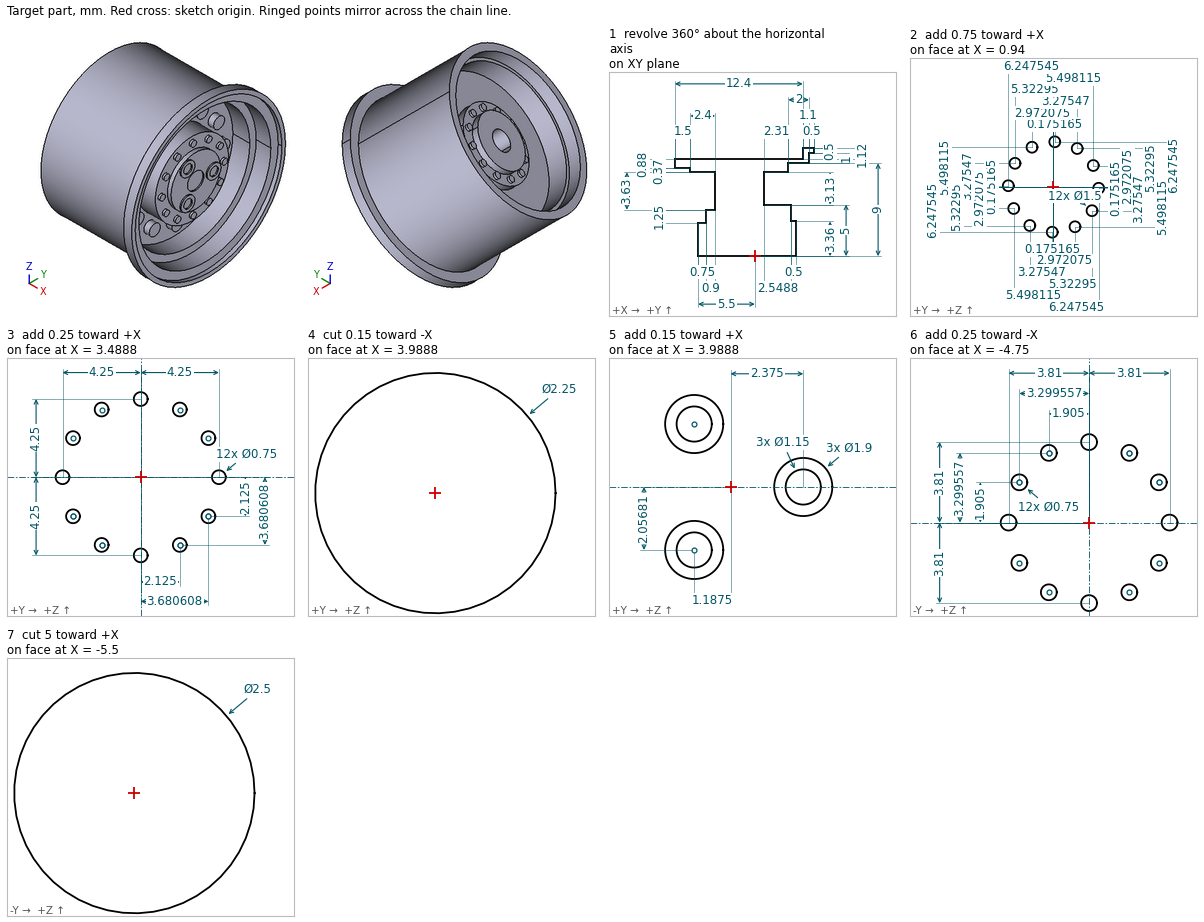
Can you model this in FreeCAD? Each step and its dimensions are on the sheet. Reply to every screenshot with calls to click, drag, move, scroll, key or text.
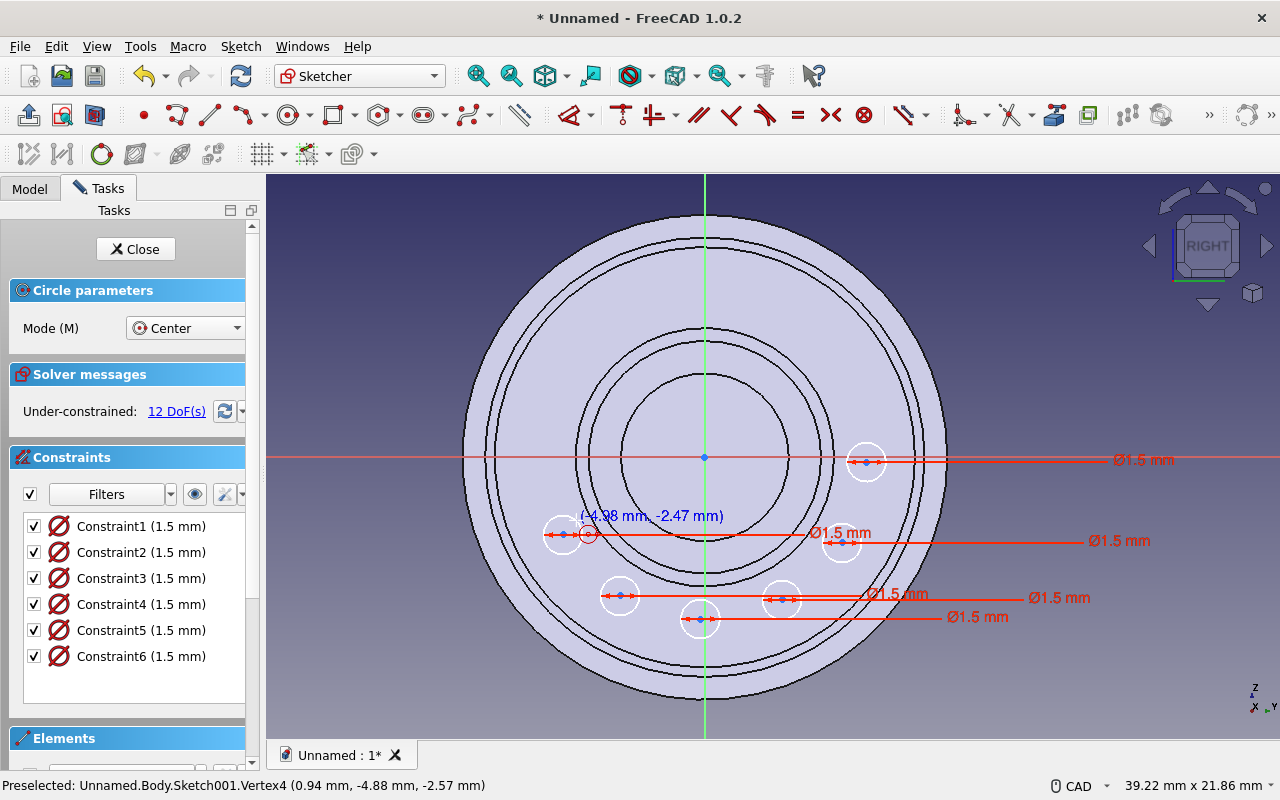
scroll(543, 453, up, 7)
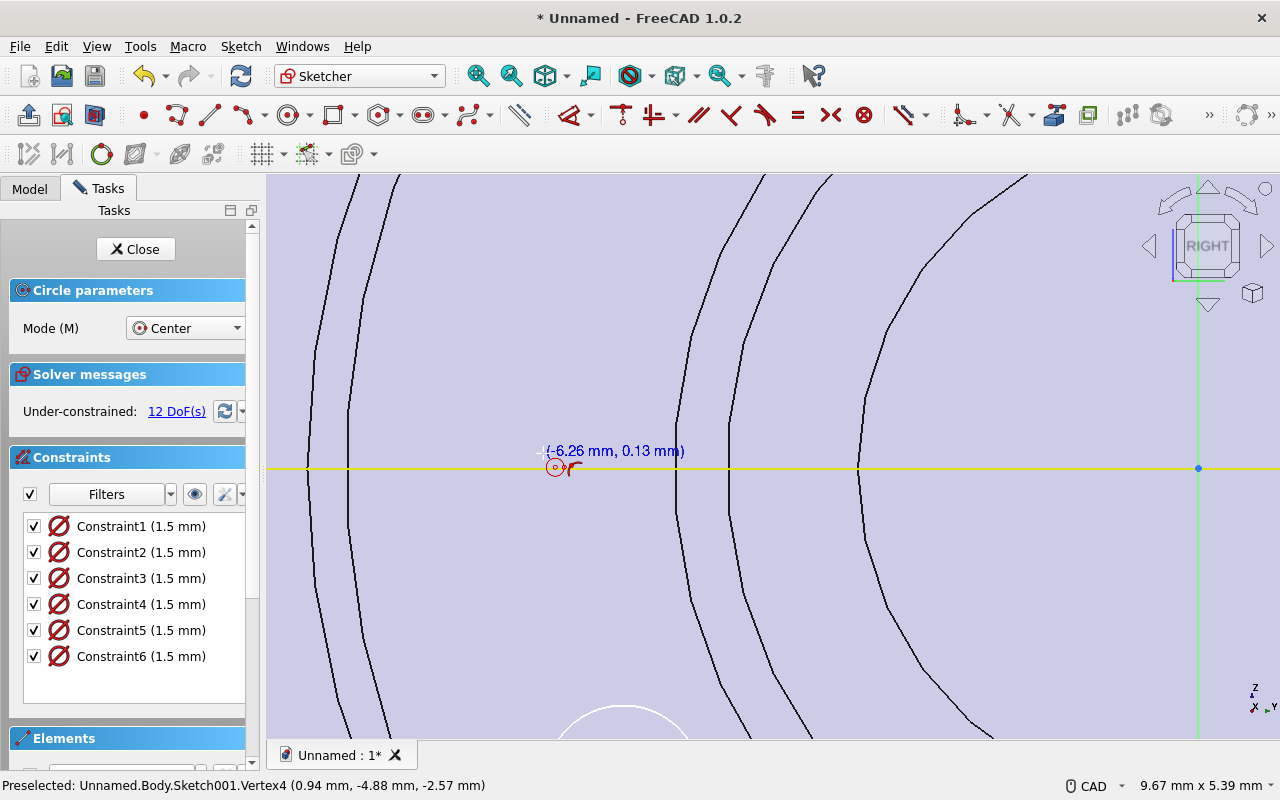
click(544, 450)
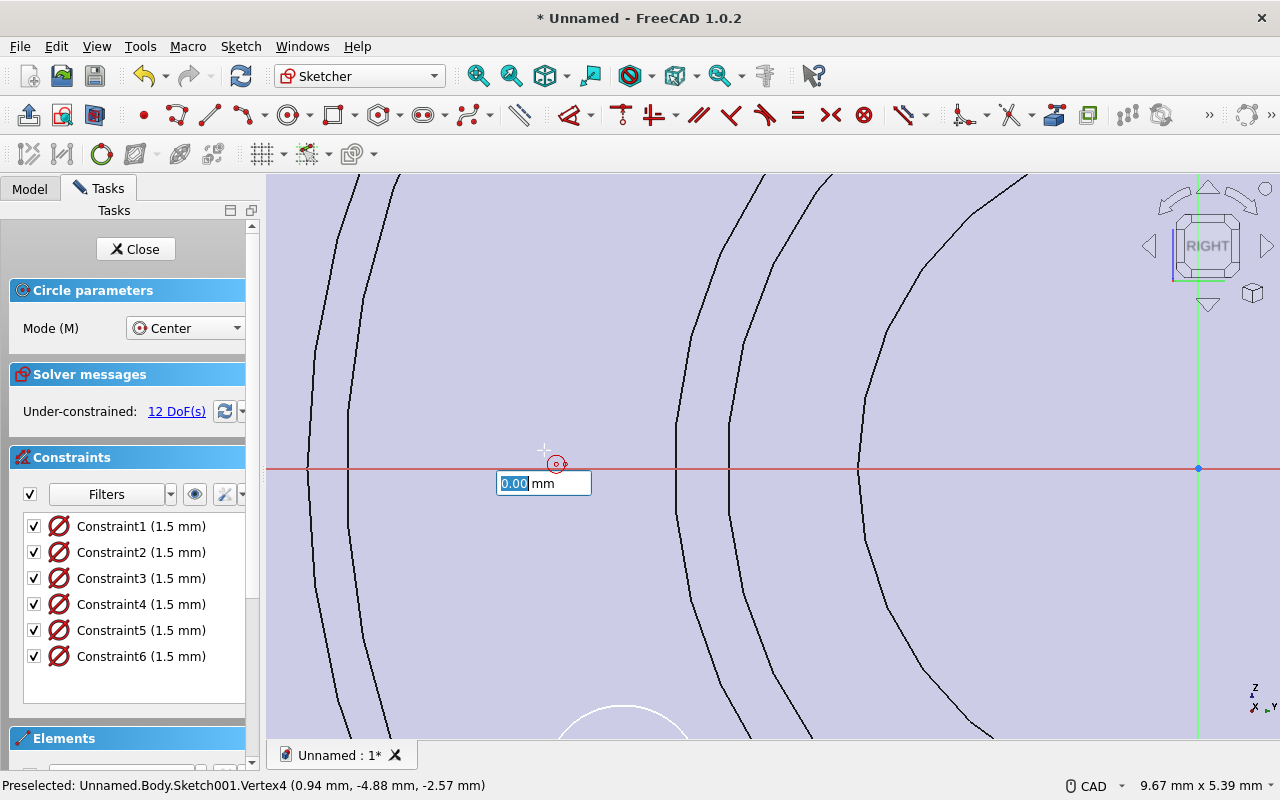
scroll(543, 452, down, 7)
move(557, 438)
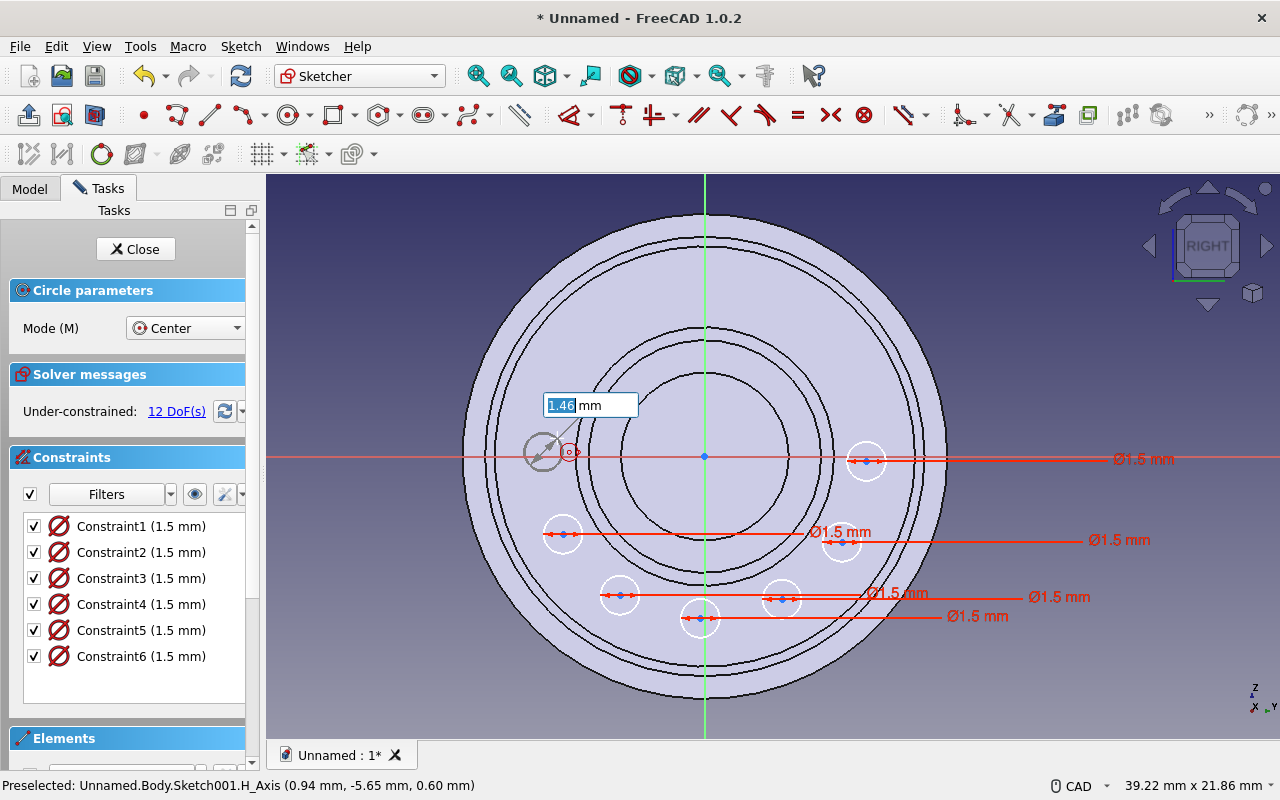
text(1.5)
key(Return)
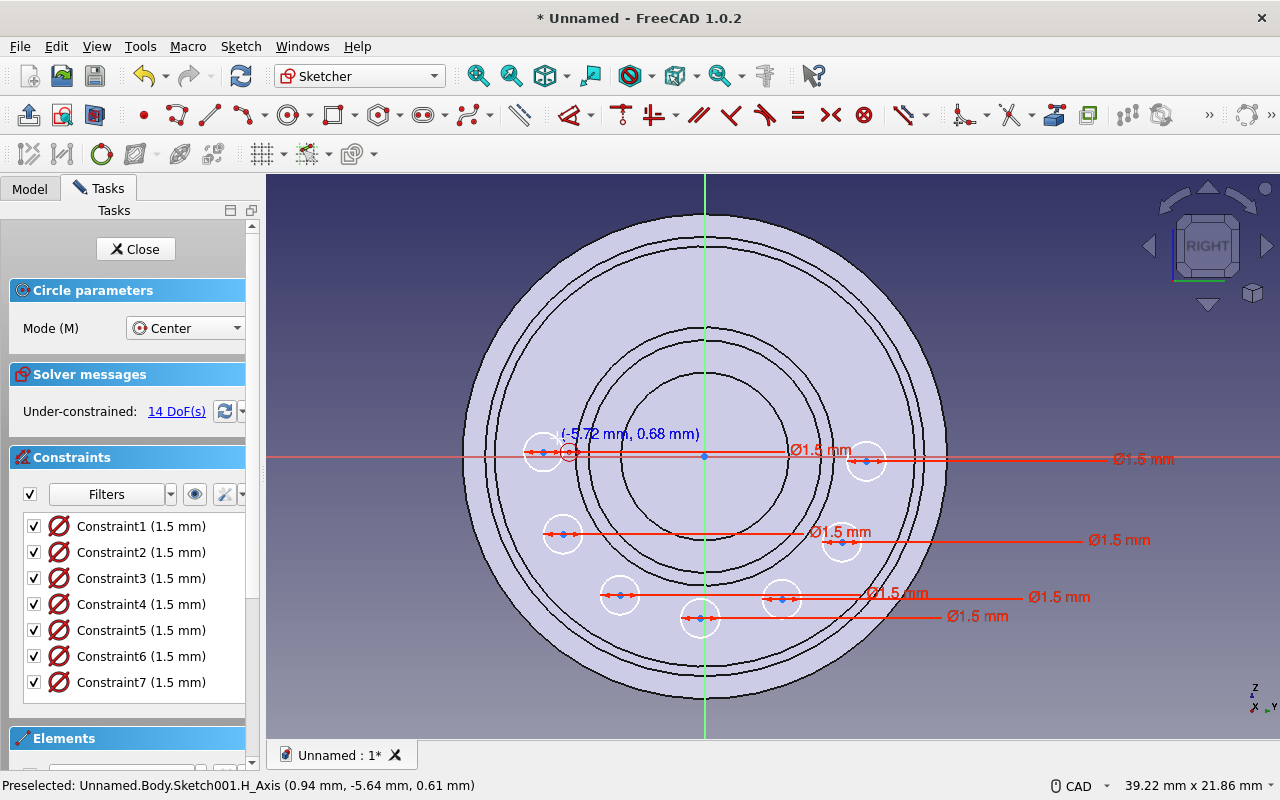
click(567, 372)
move(581, 358)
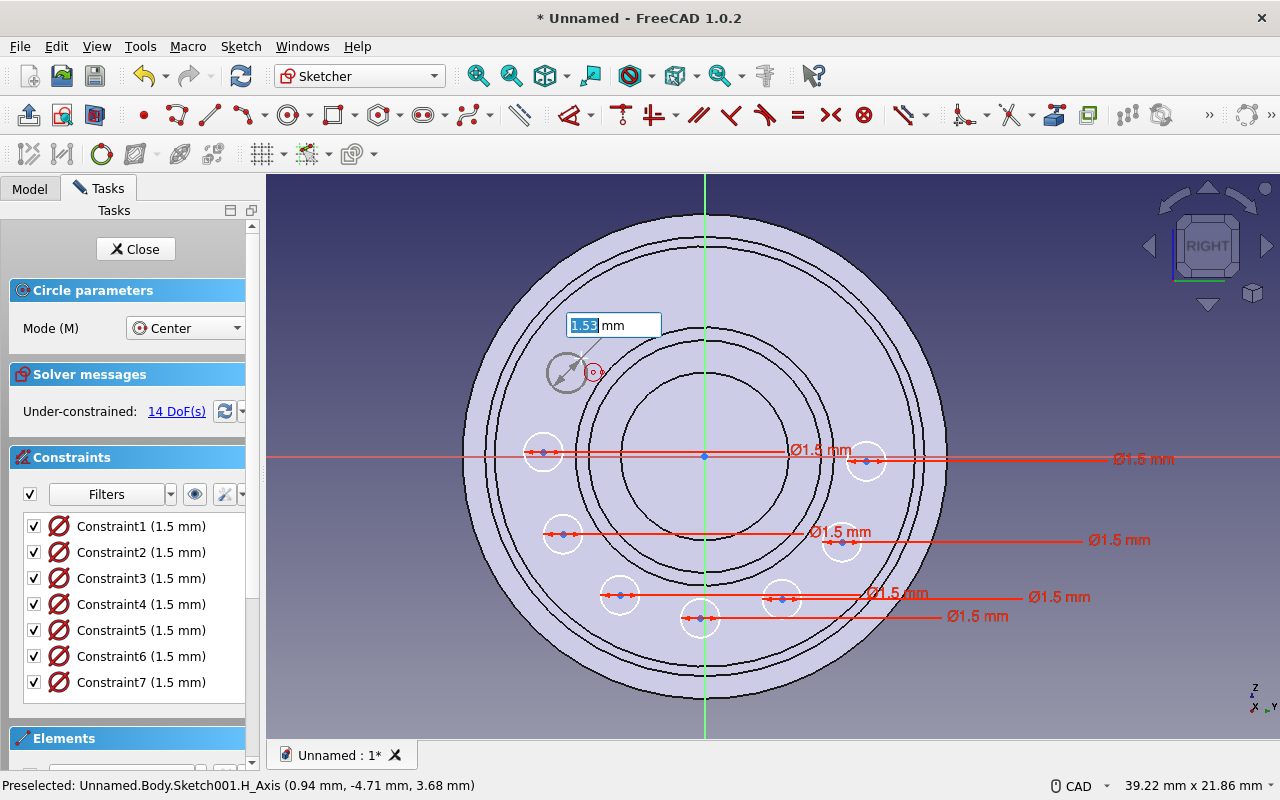
text(1.5)
key(Return)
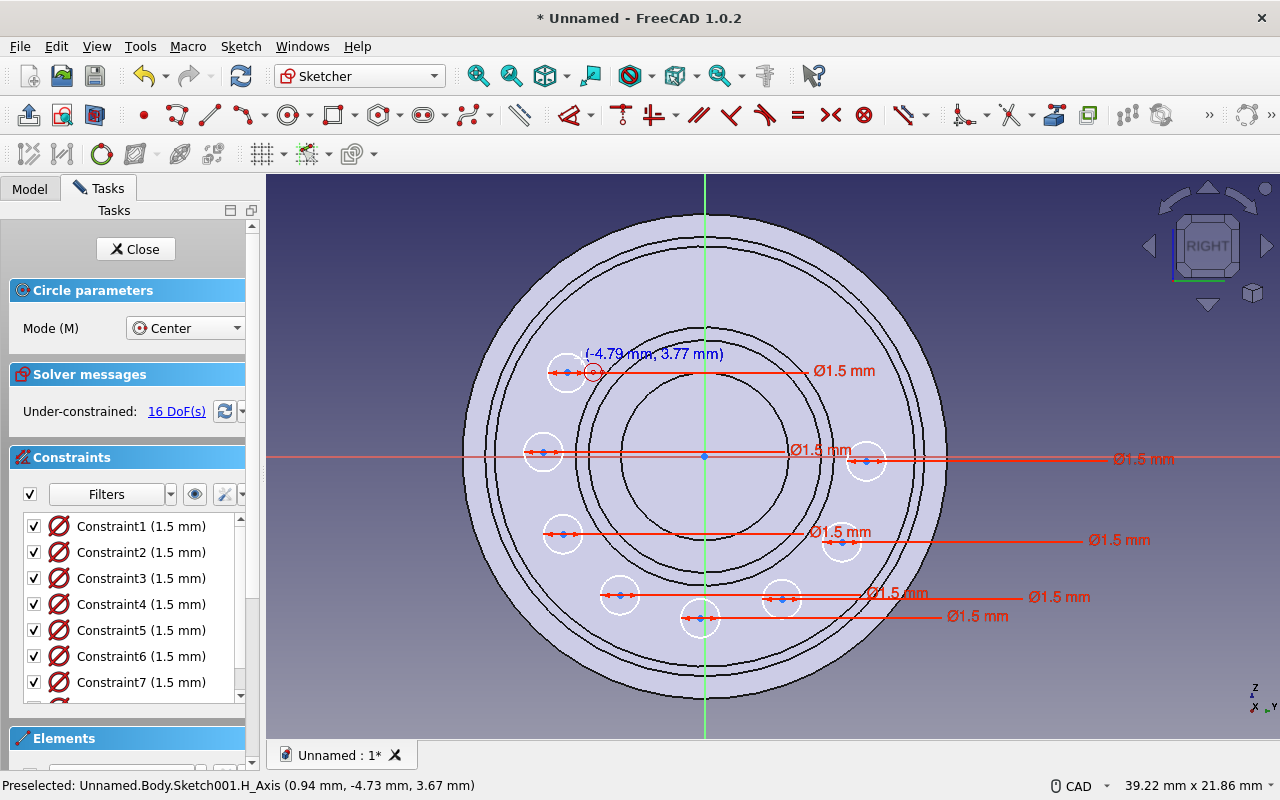
click(628, 314)
move(642, 301)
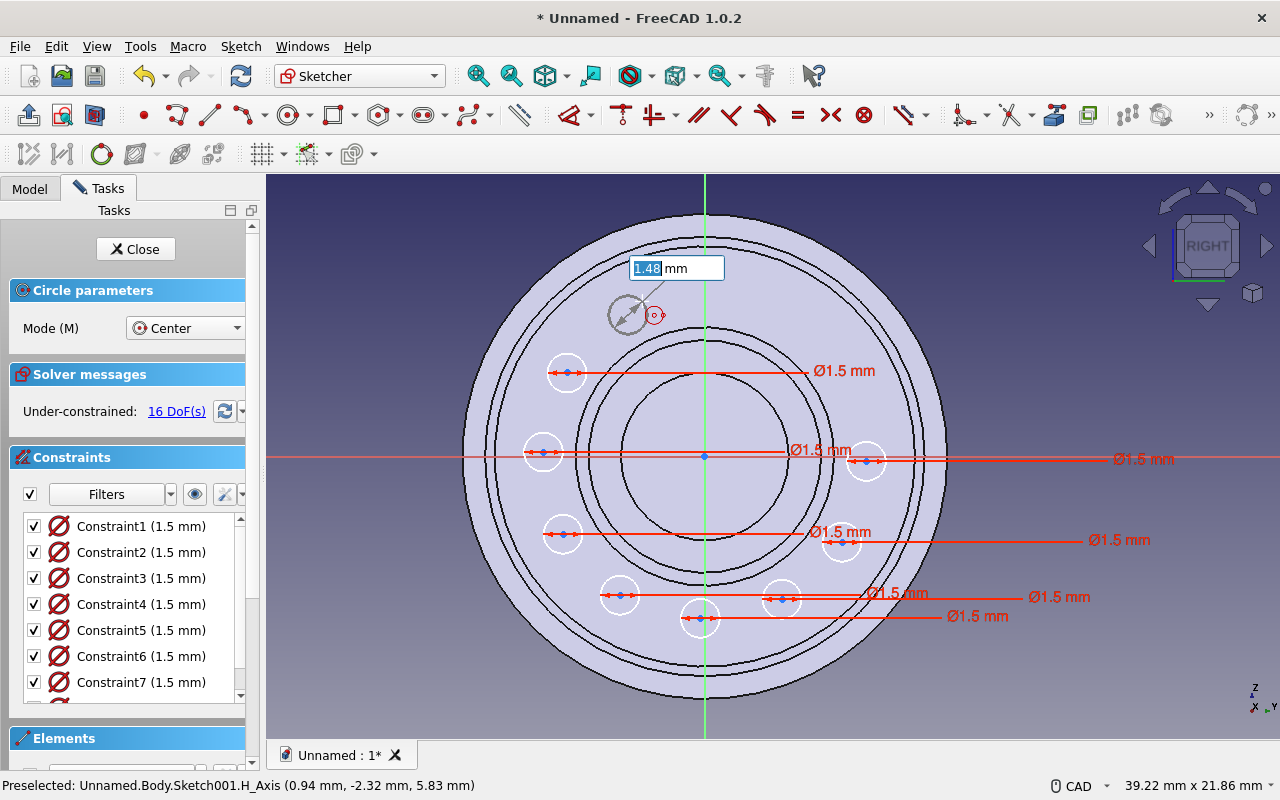
text(1.5)
key(Return)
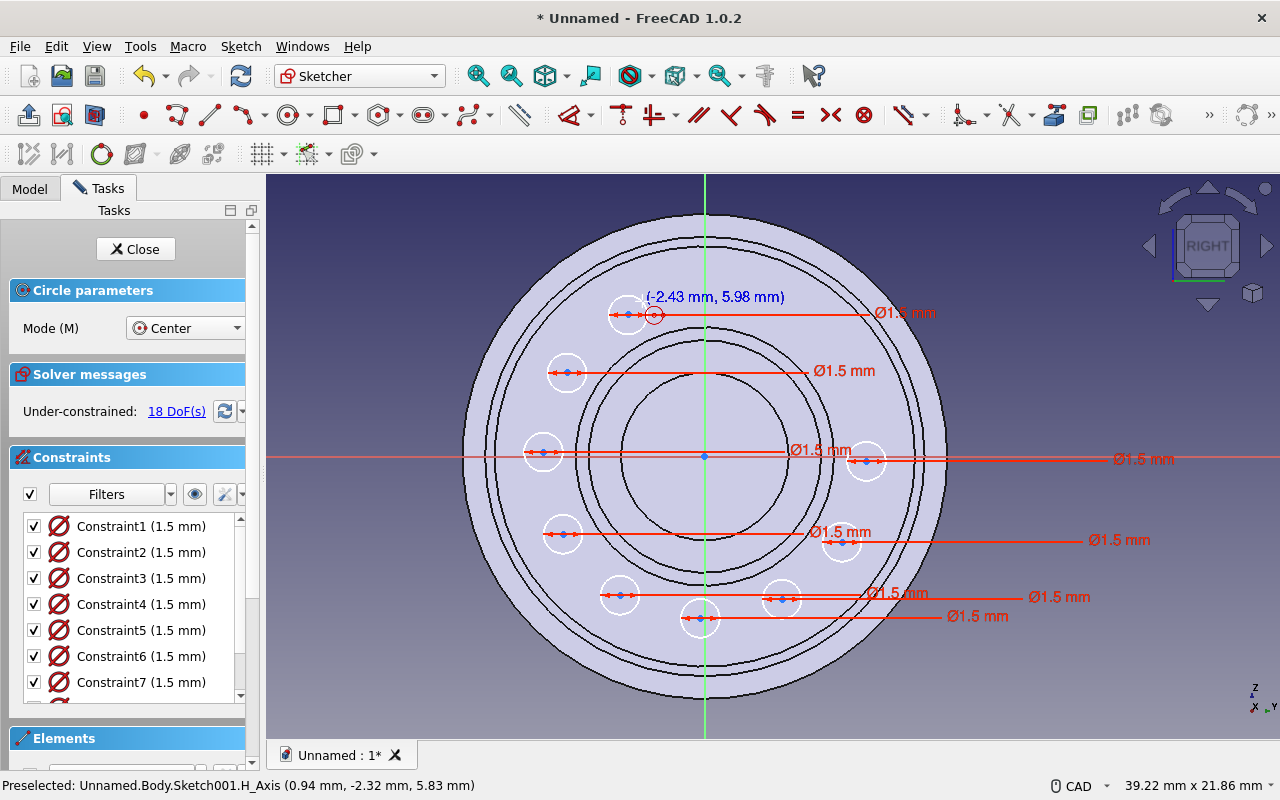
scroll(709, 295, up, 7)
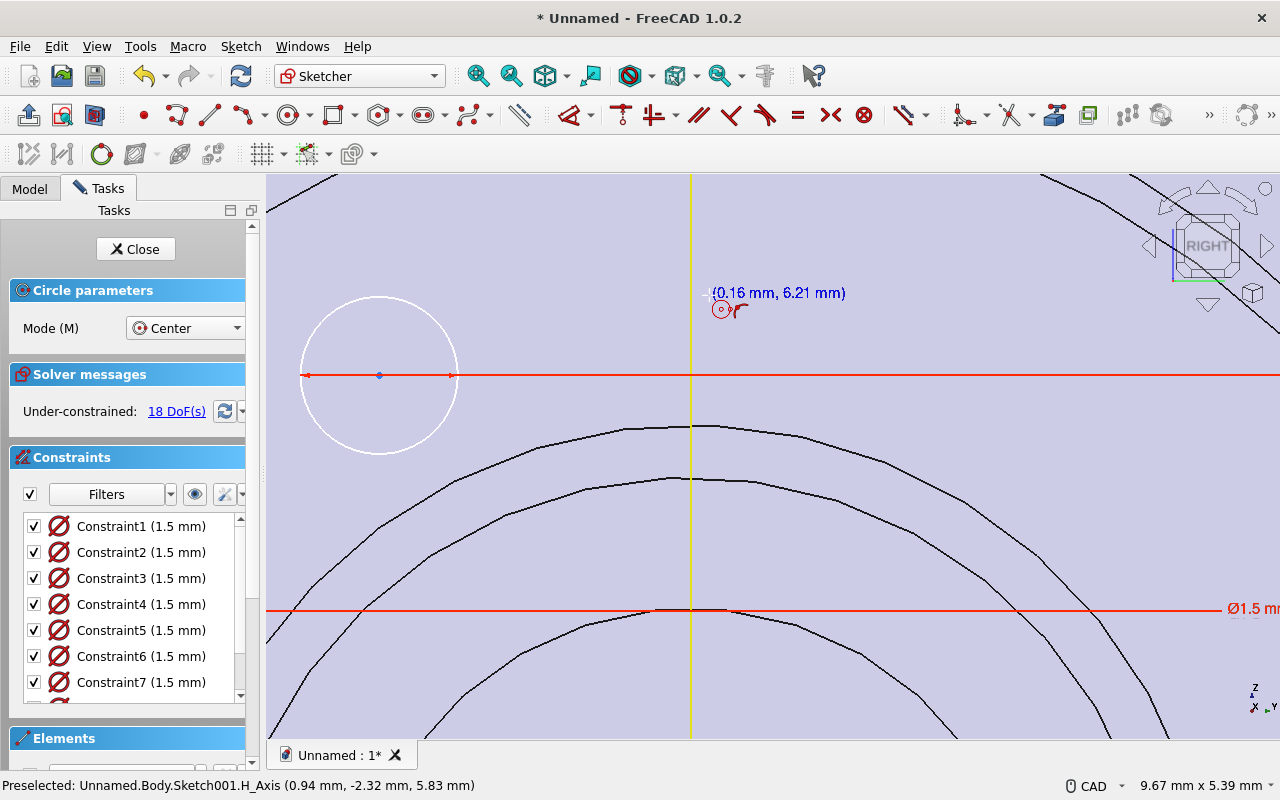
click(709, 294)